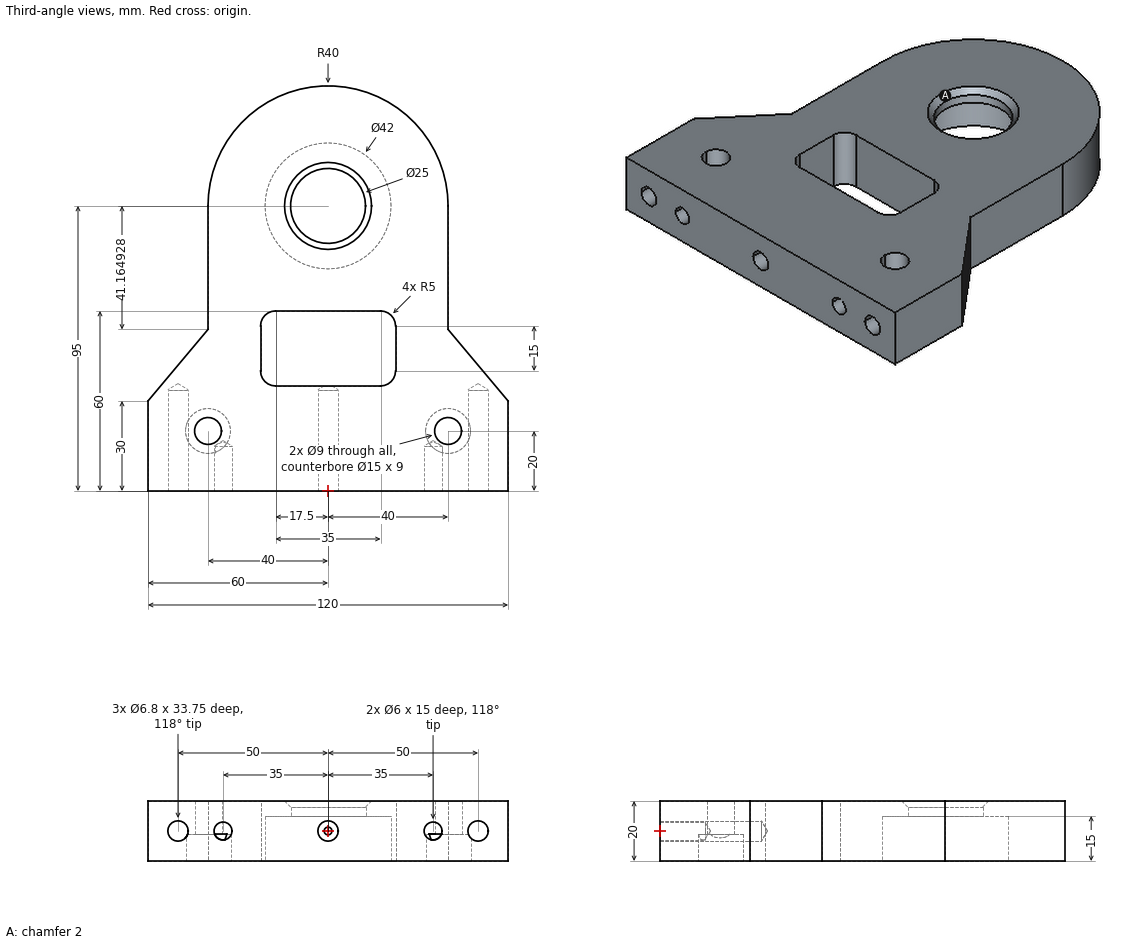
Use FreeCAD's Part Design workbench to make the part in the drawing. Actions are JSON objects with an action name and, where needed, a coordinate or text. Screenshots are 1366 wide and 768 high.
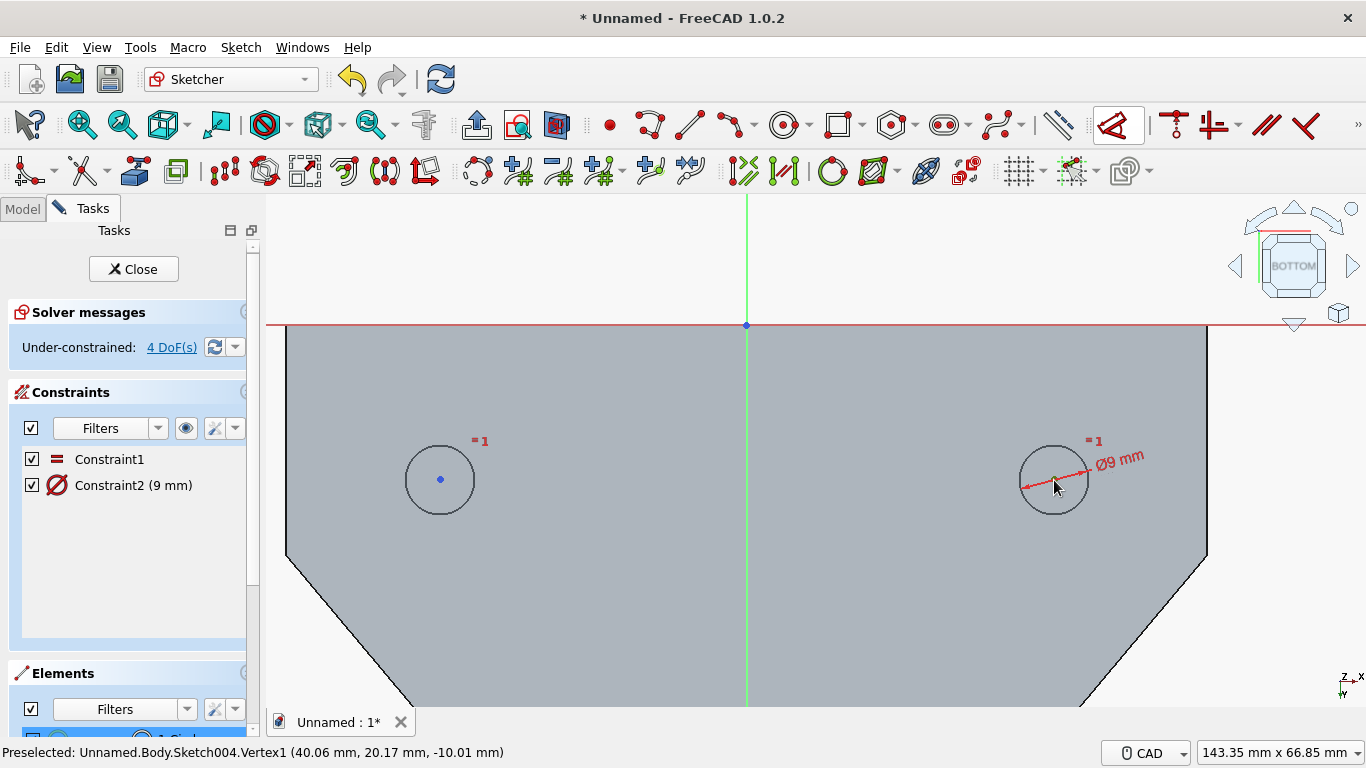
{"action": "left_click", "coordinate": [1138, 126]}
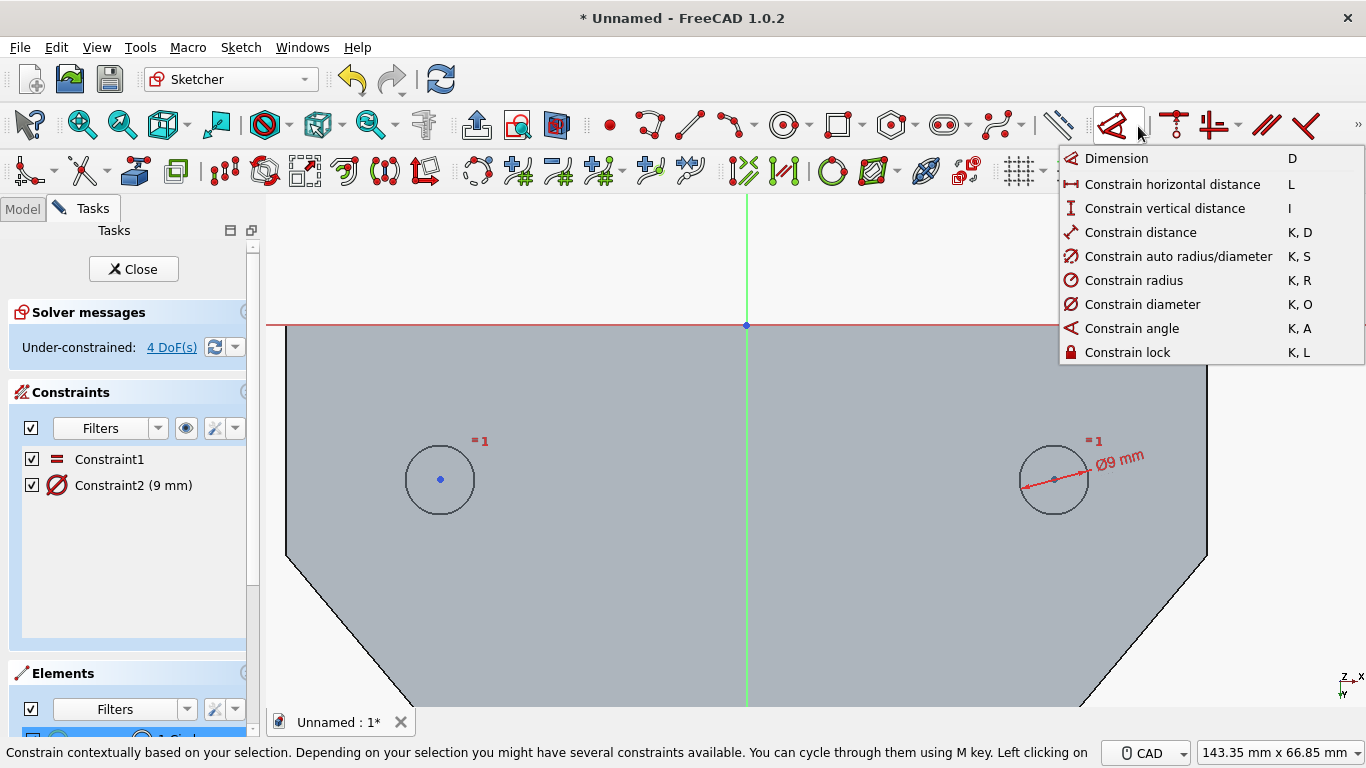
{"action": "left_click", "coordinate": [1212, 184]}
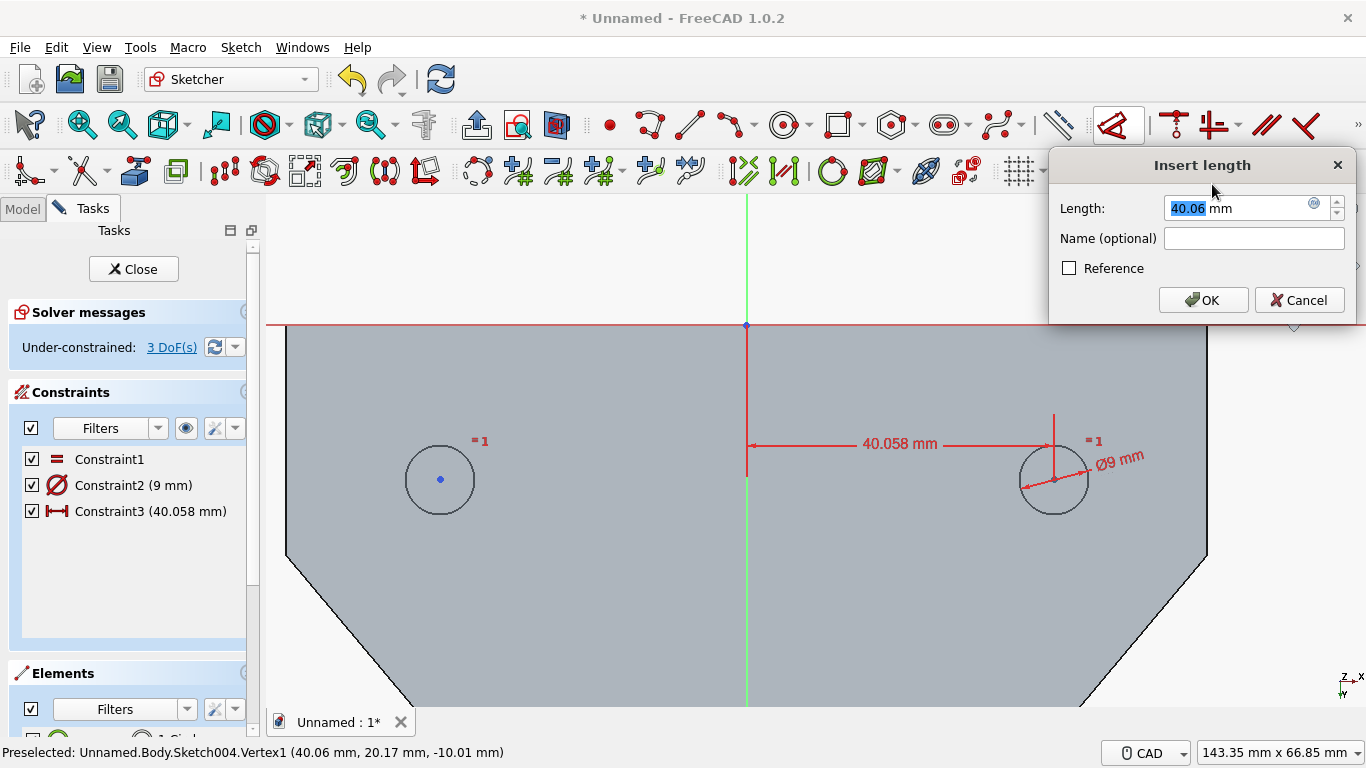
{"action": "type", "text": "40"}
{"action": "key", "text": "Return"}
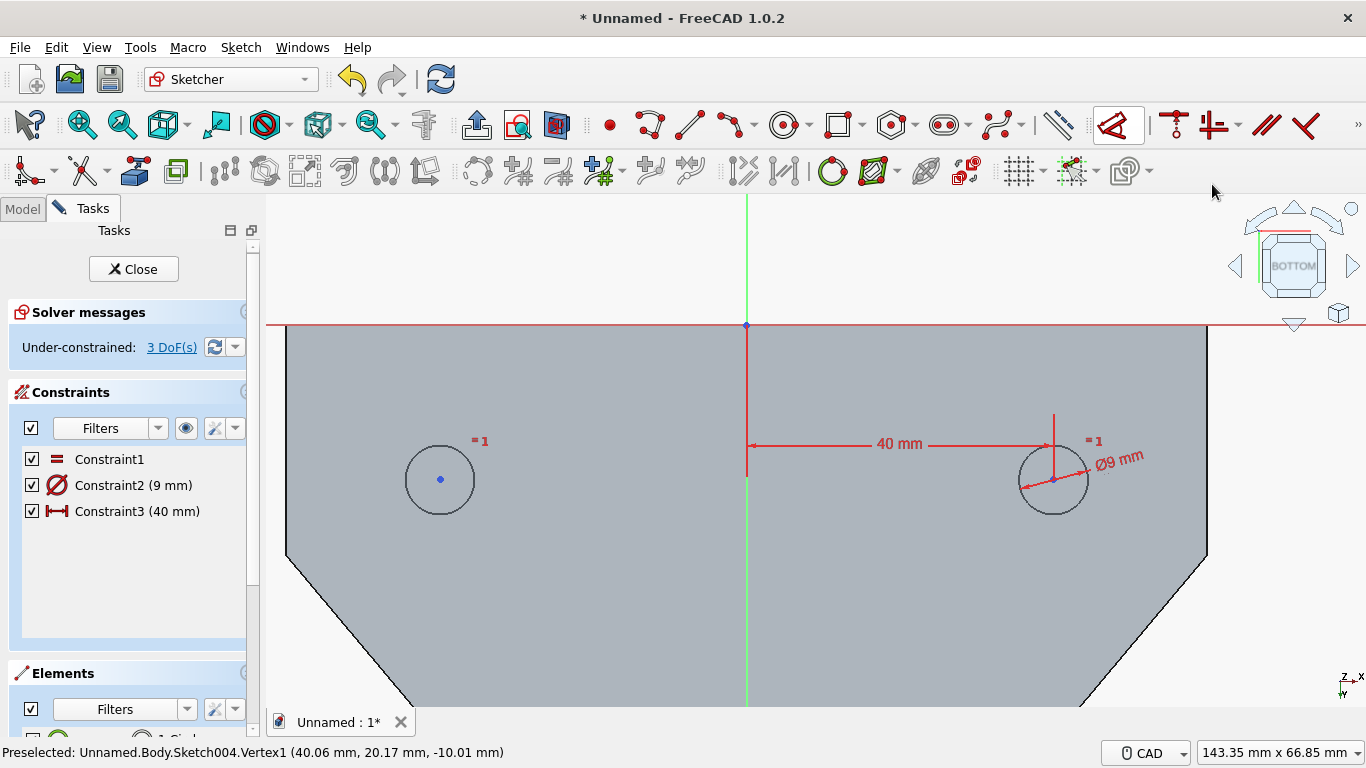
{"action": "left_click", "coordinate": [1054, 480]}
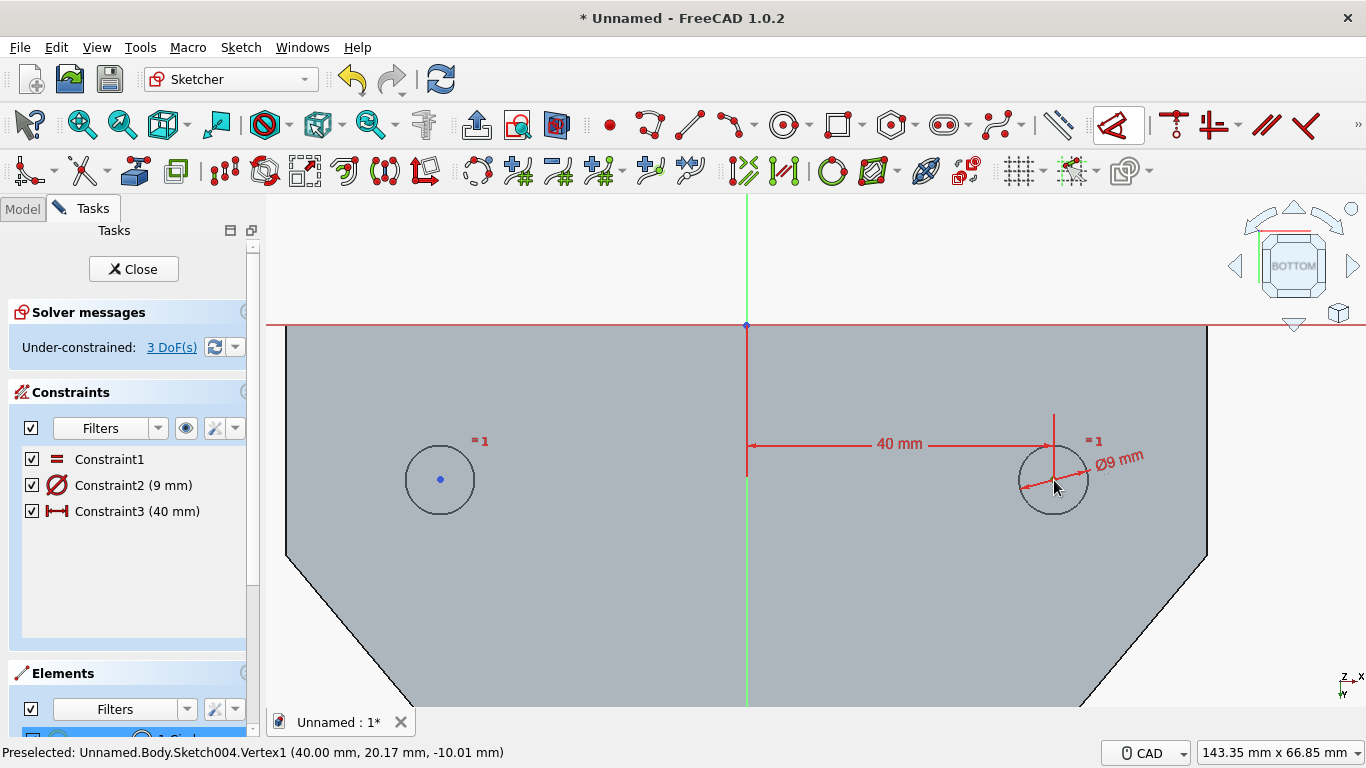
{"action": "left_click", "coordinate": [1138, 126]}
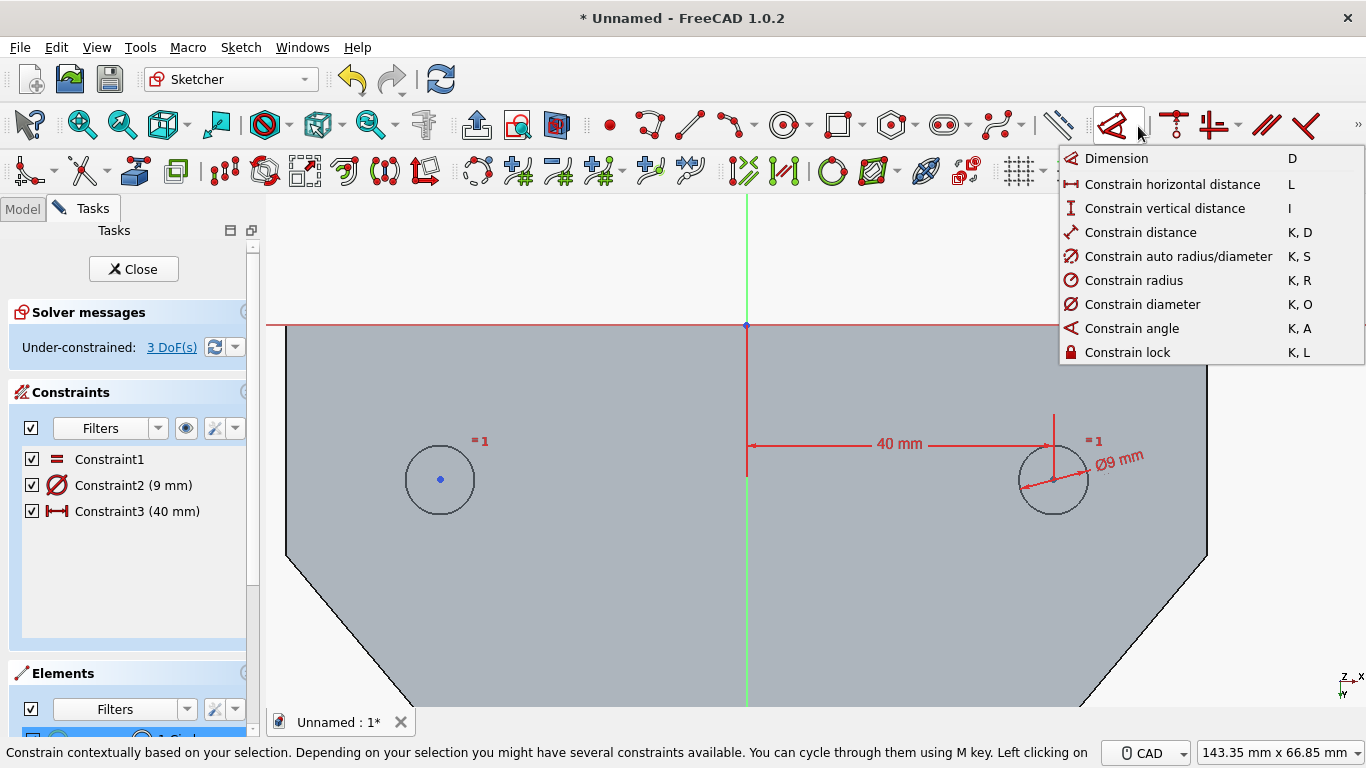
{"action": "left_click", "coordinate": [1212, 208]}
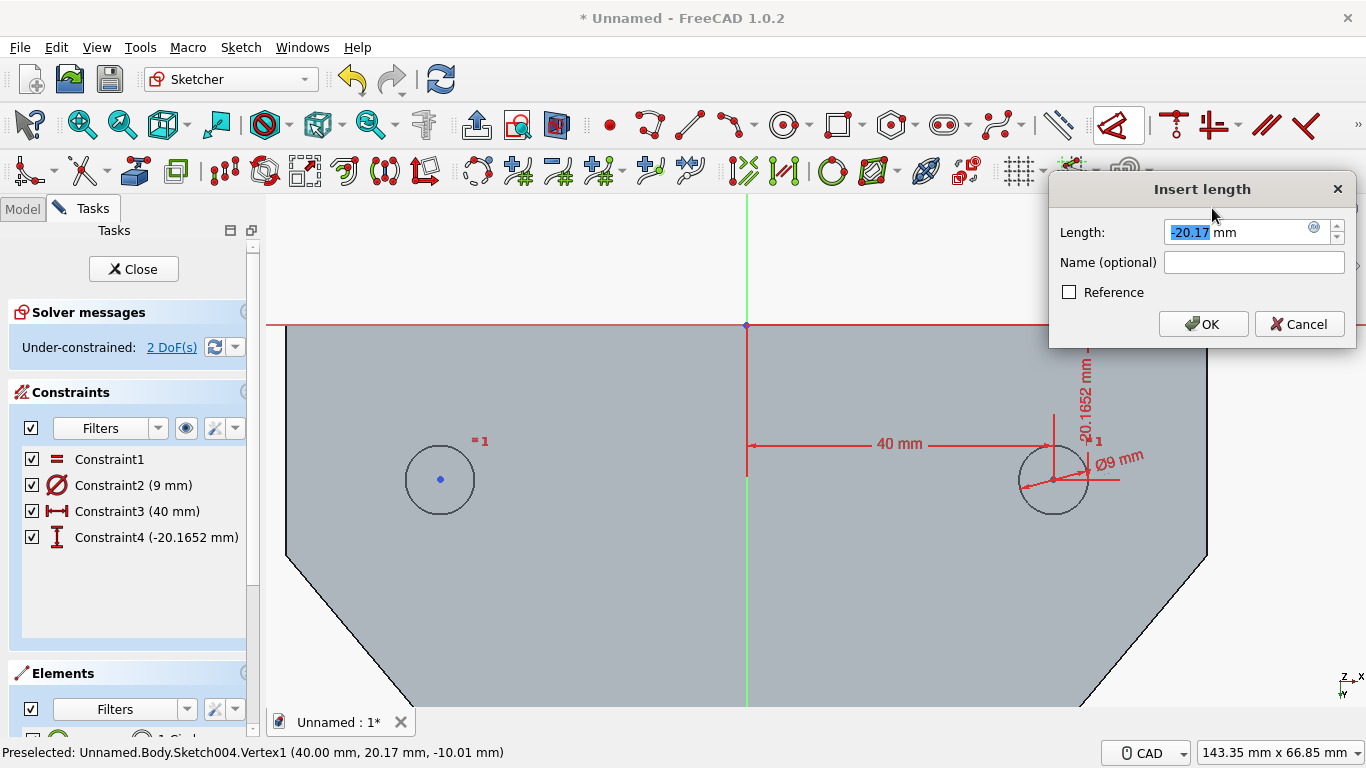
{"action": "type", "text": "-20"}
{"action": "key", "text": "Return"}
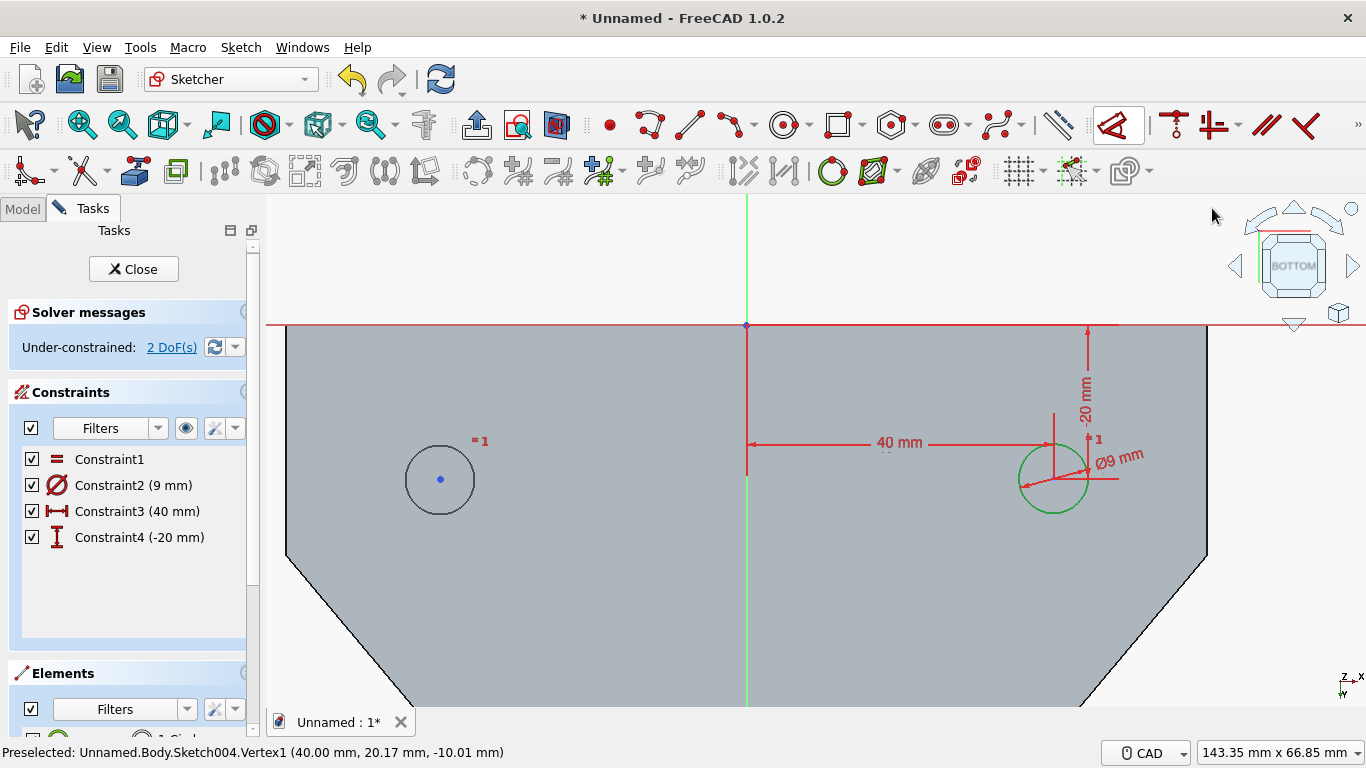
{"action": "left_click", "coordinate": [440, 480]}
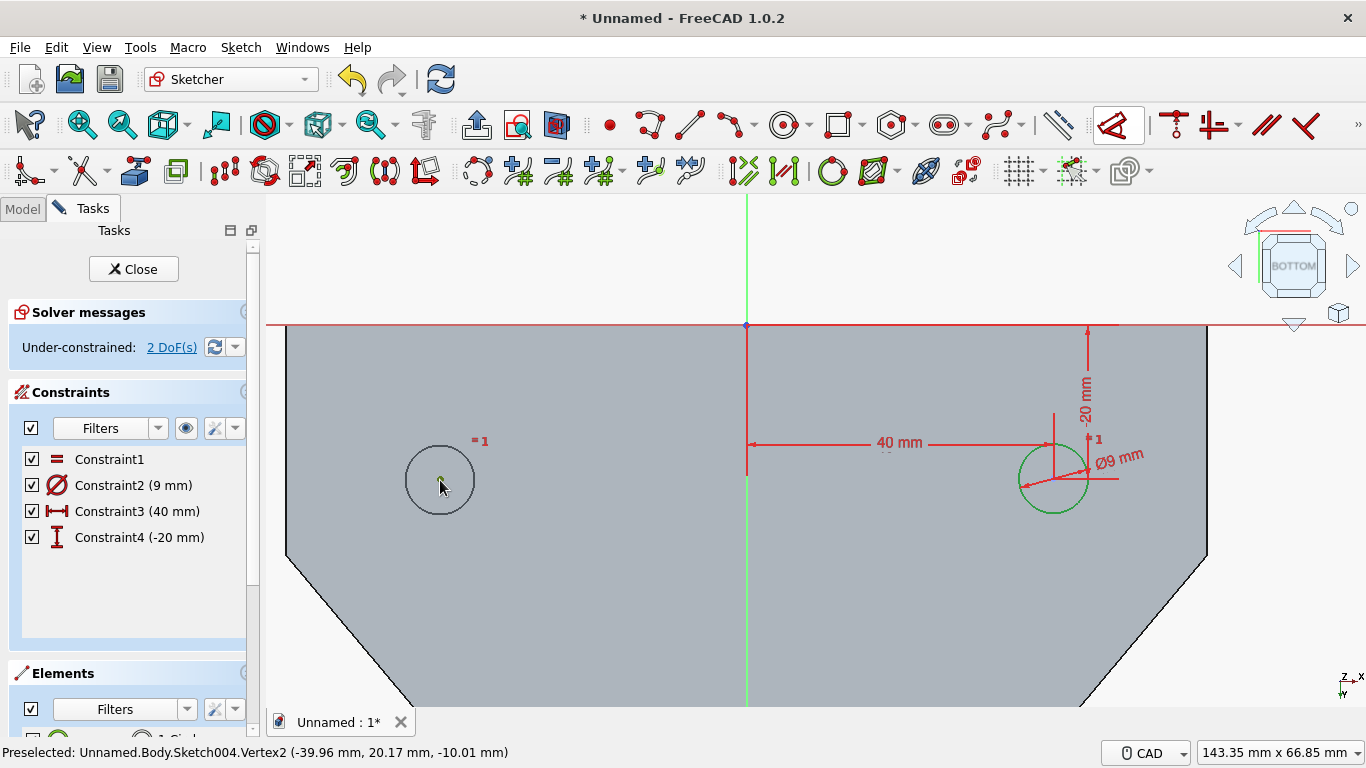
{"action": "left_click", "coordinate": [1138, 126]}